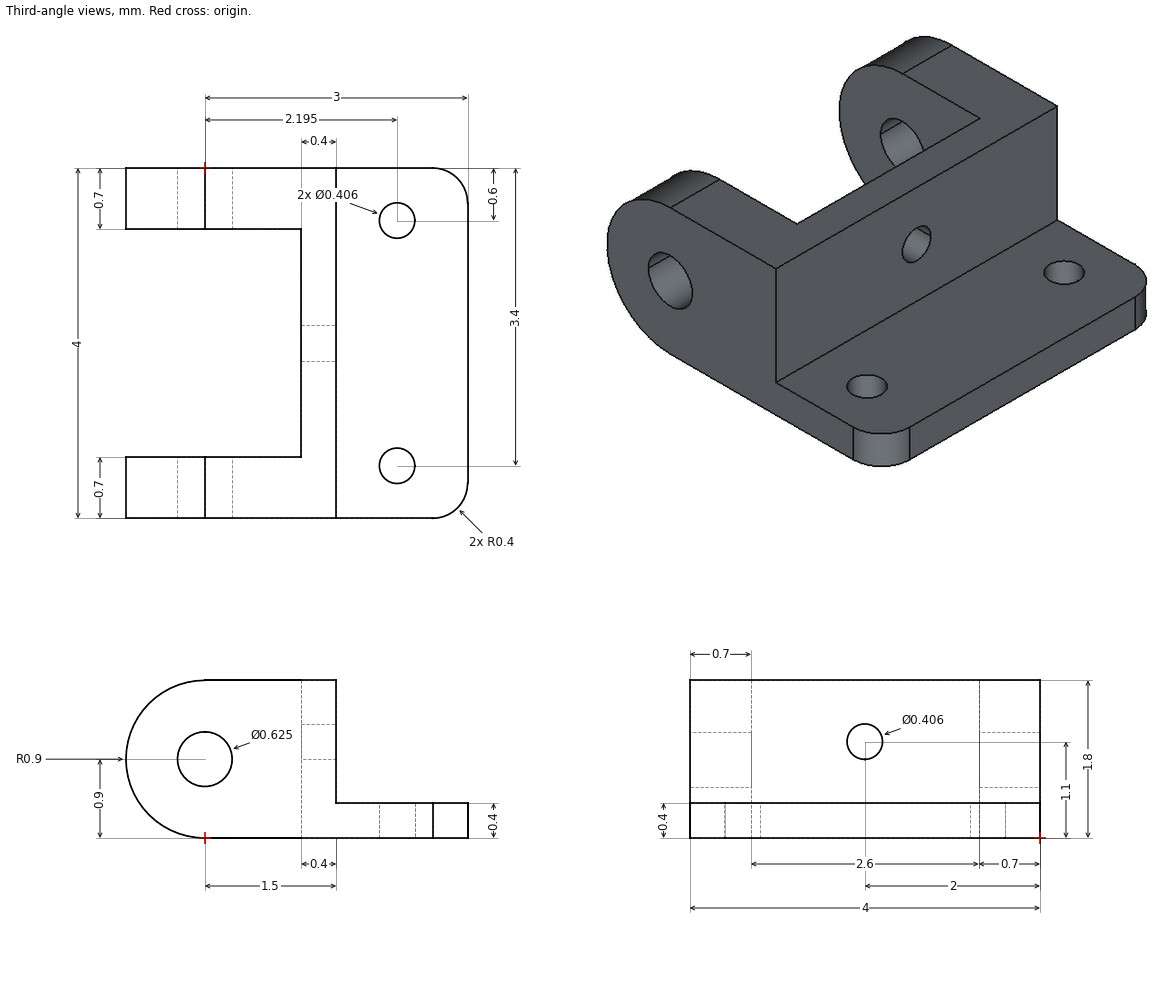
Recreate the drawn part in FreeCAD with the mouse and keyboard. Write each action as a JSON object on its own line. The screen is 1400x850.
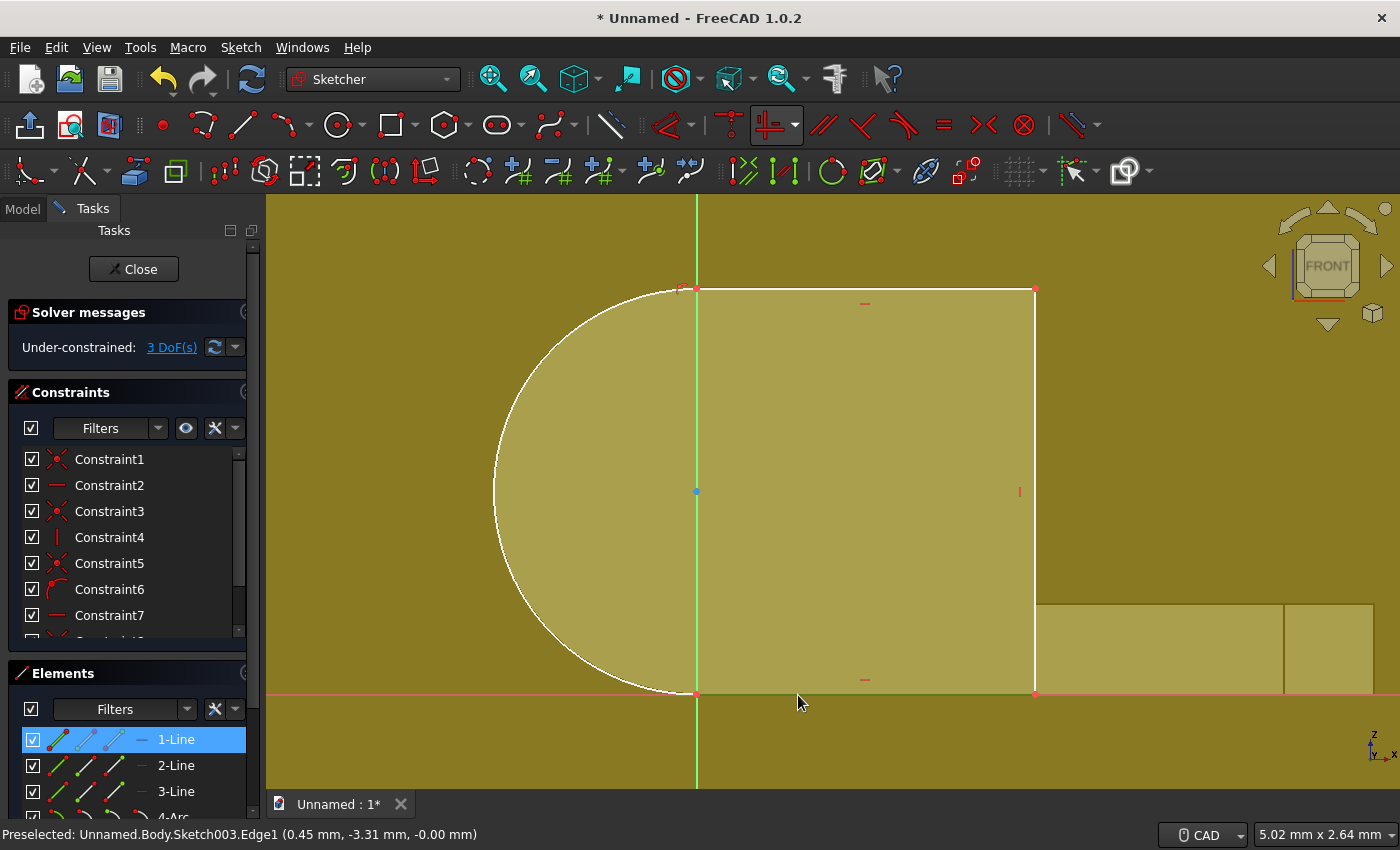
{"action": "left_click", "coordinate": [533, 373]}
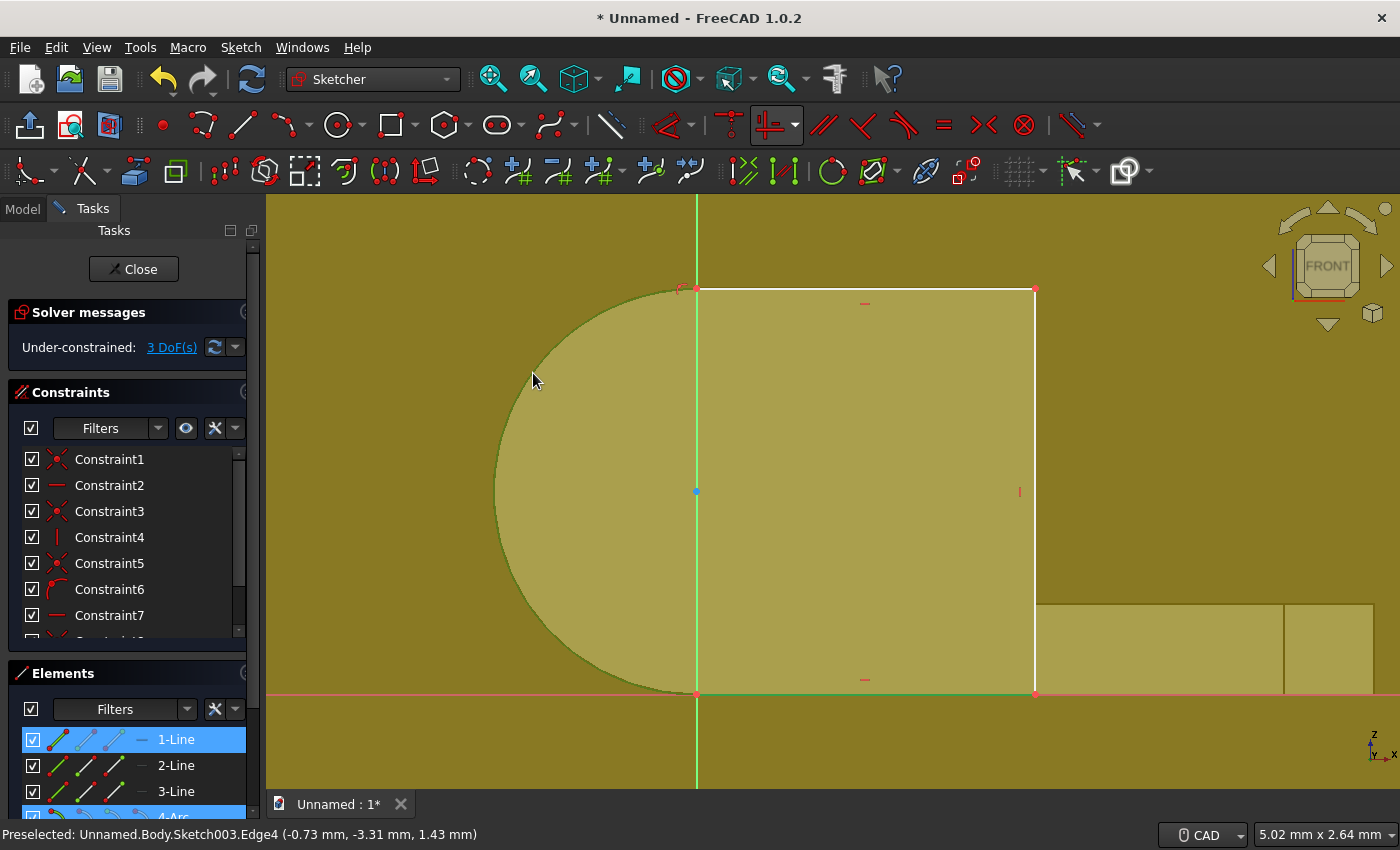
{"action": "key", "text": "t"}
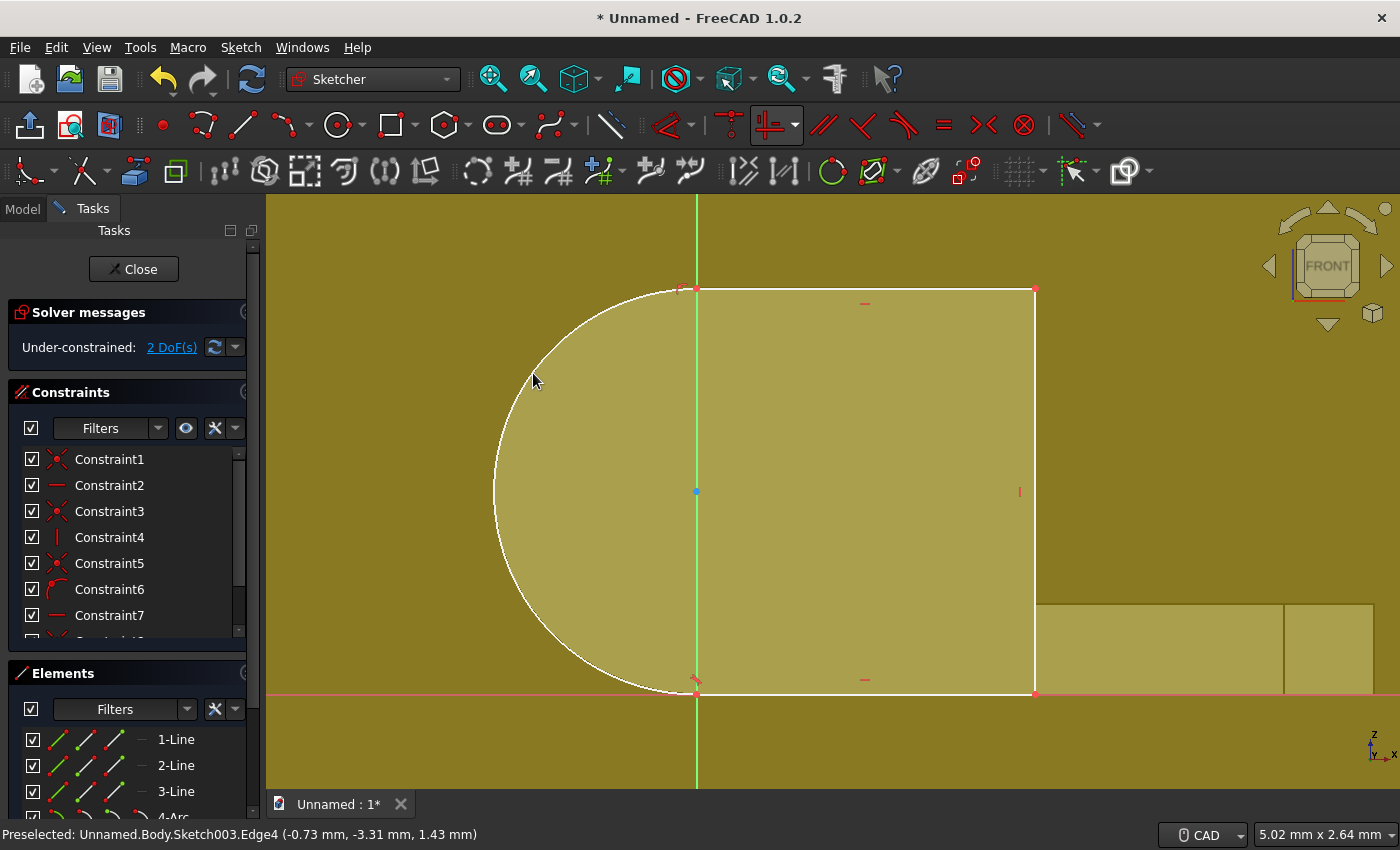
{"action": "key", "text": "d"}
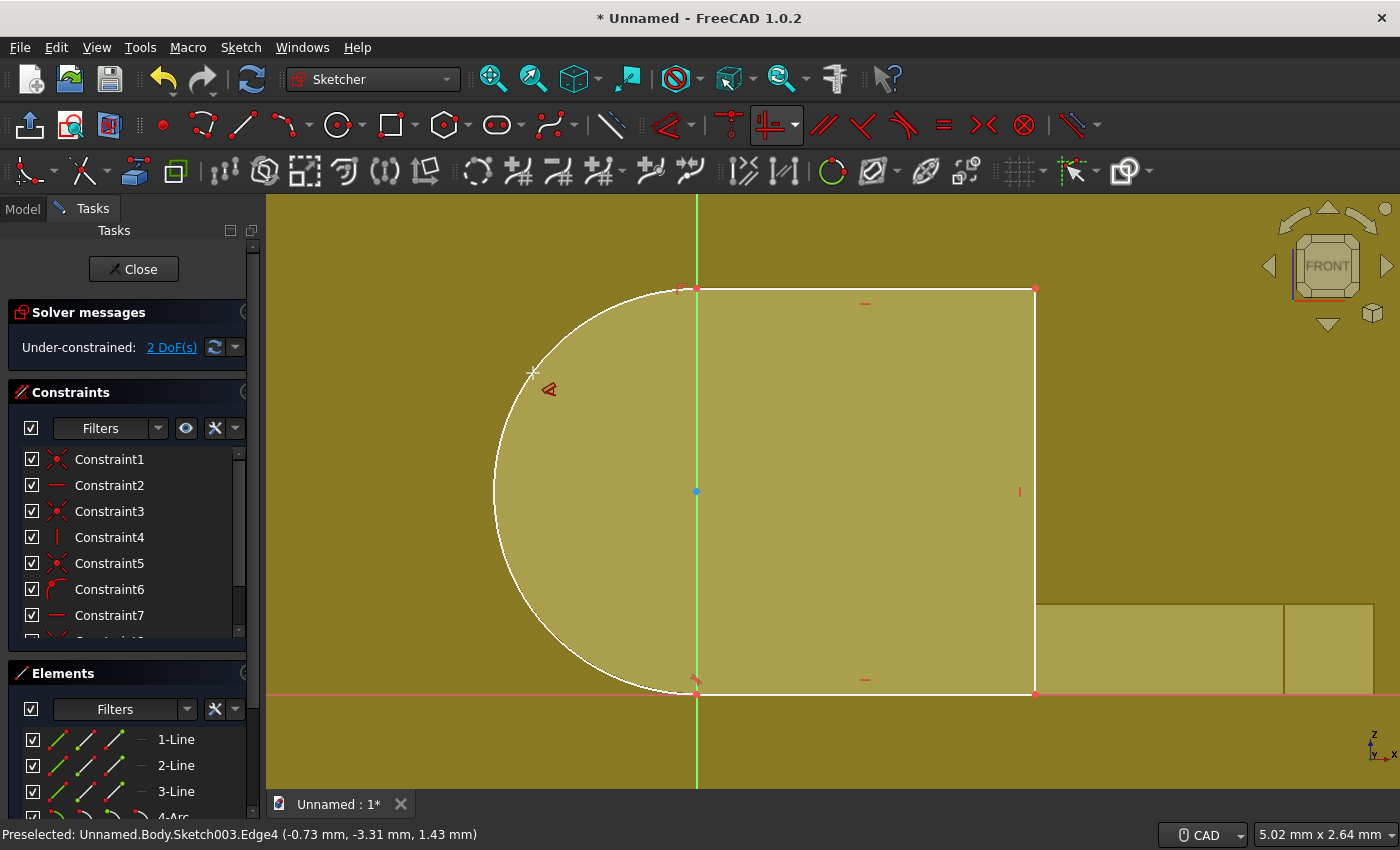
{"action": "left_click", "coordinate": [533, 373]}
{"action": "left_click", "coordinate": [507, 354]}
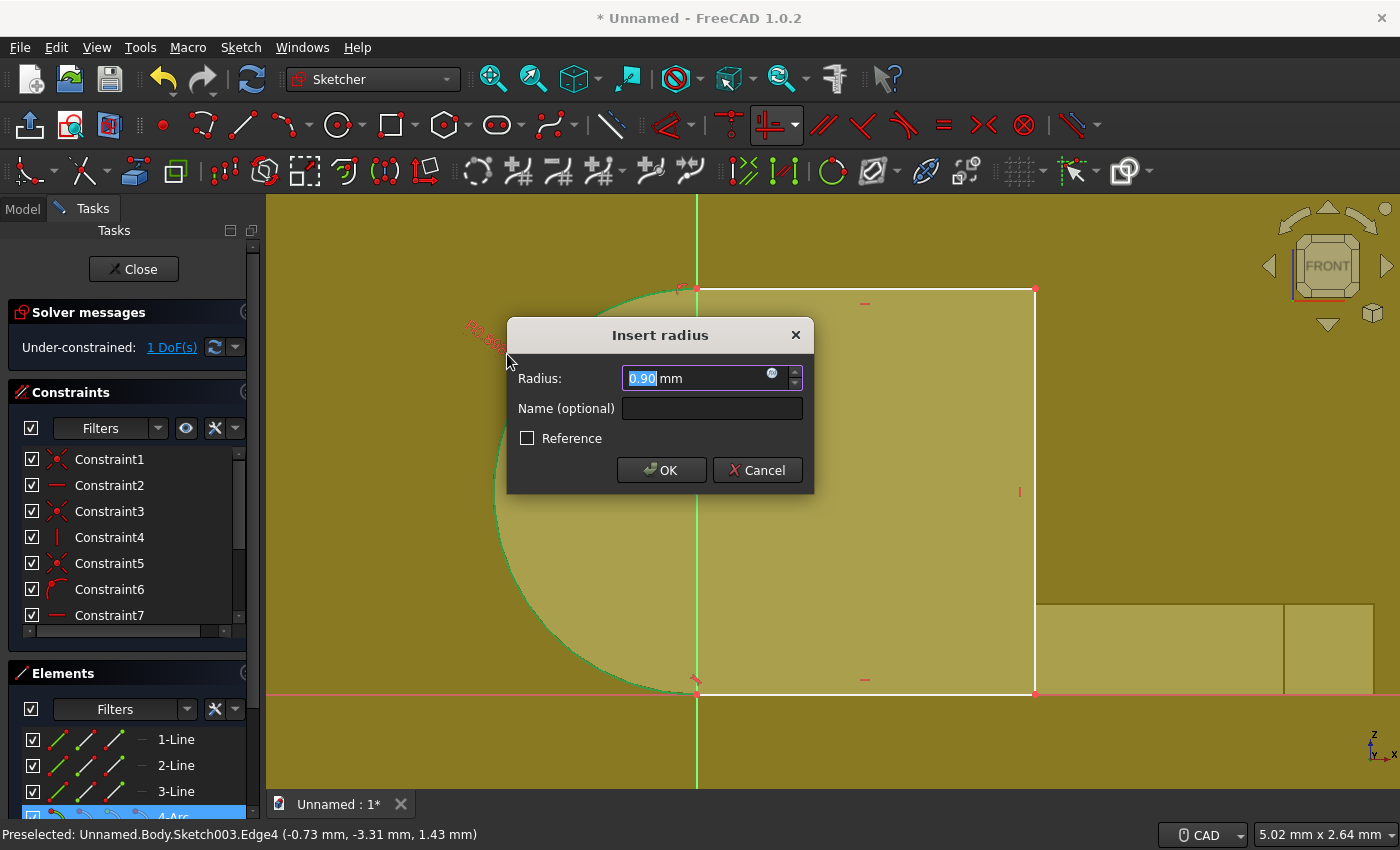
{"action": "type", "text": "0.9"}
{"action": "key", "text": "Return"}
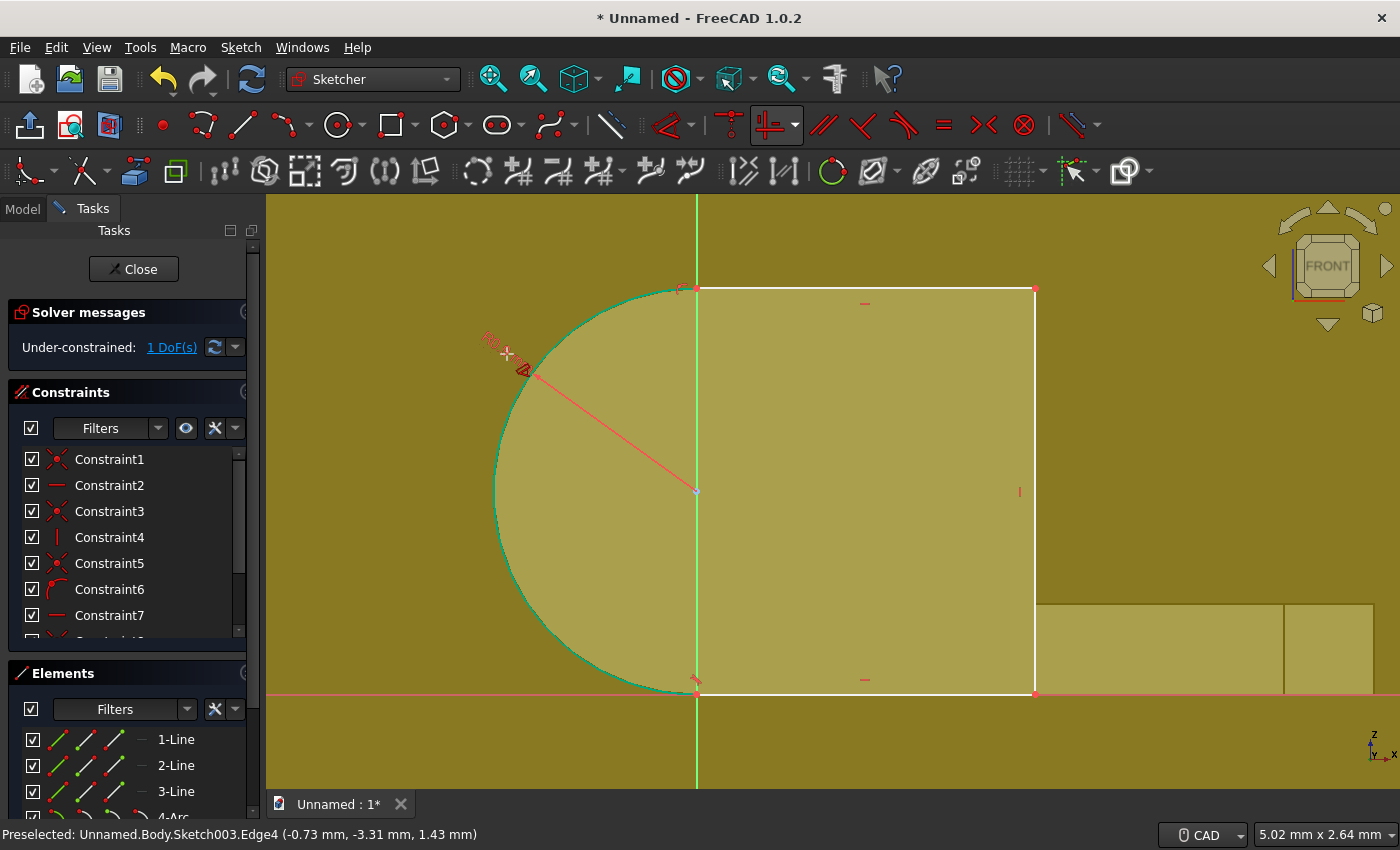
{"action": "left_click", "coordinate": [798, 695]}
{"action": "left_click", "coordinate": [866, 729]}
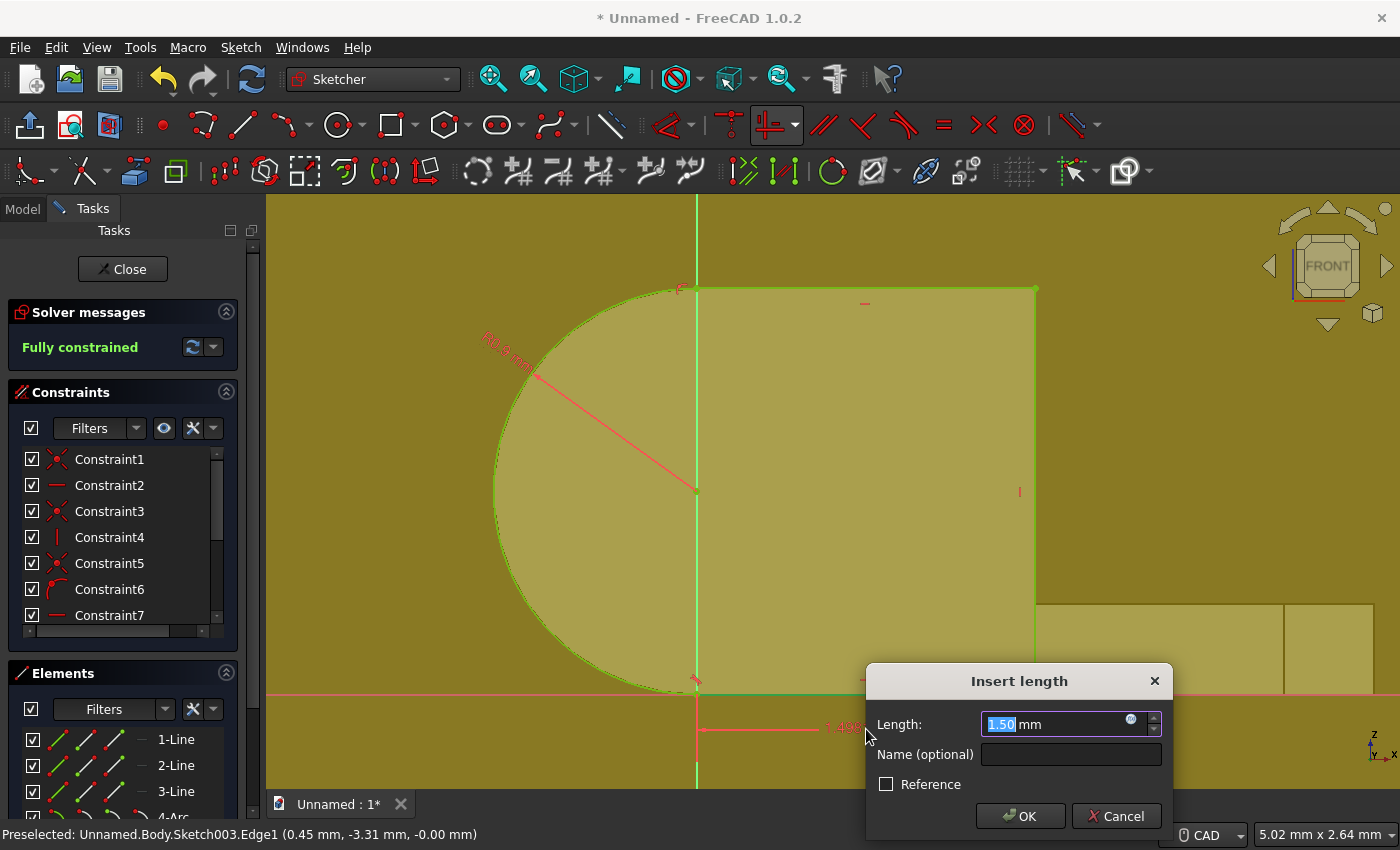
{"action": "type", "text": "1.5"}
{"action": "key", "text": "Return"}
{"action": "key", "text": "Escape"}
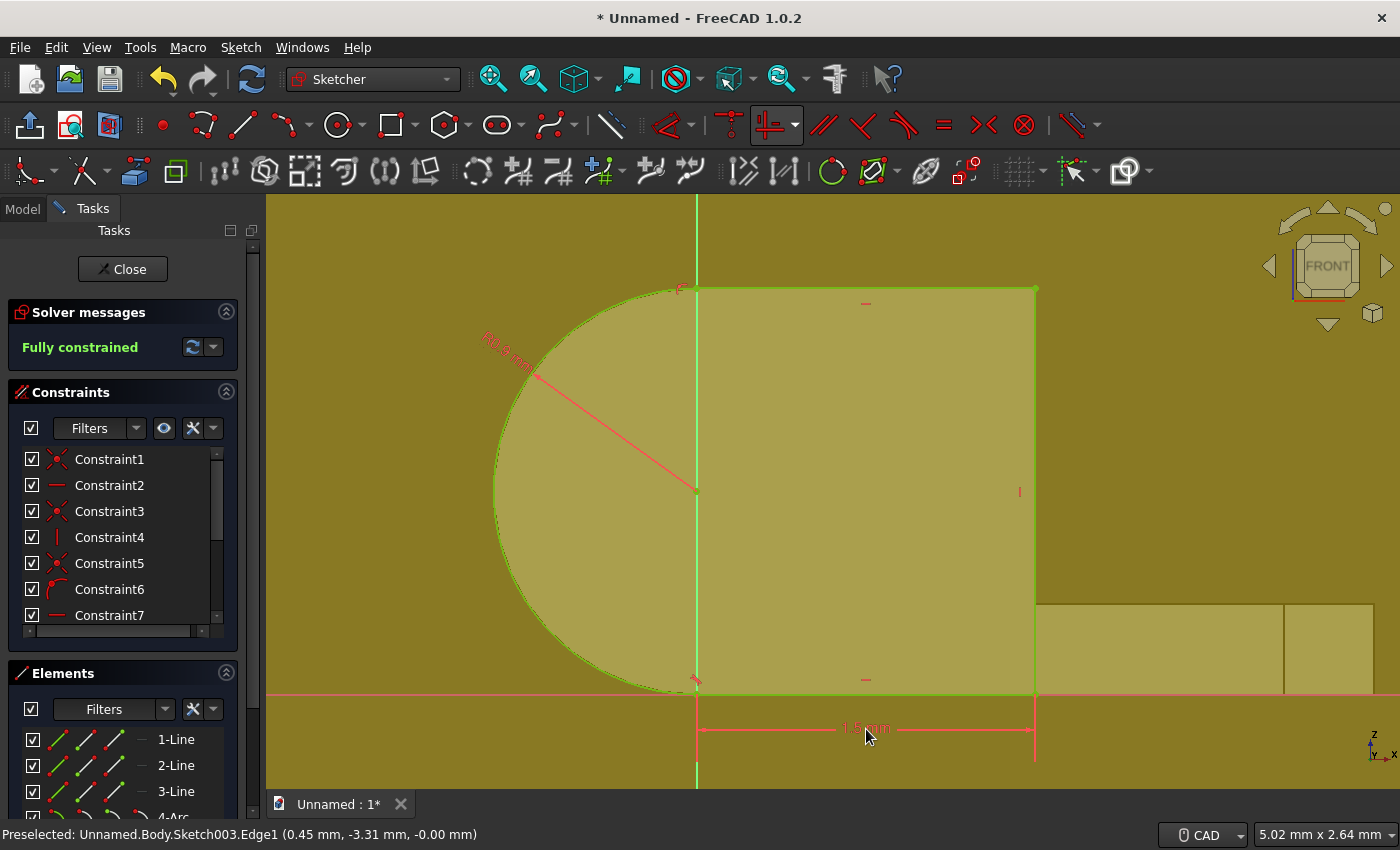
{"action": "left_click", "coordinate": [123, 269]}